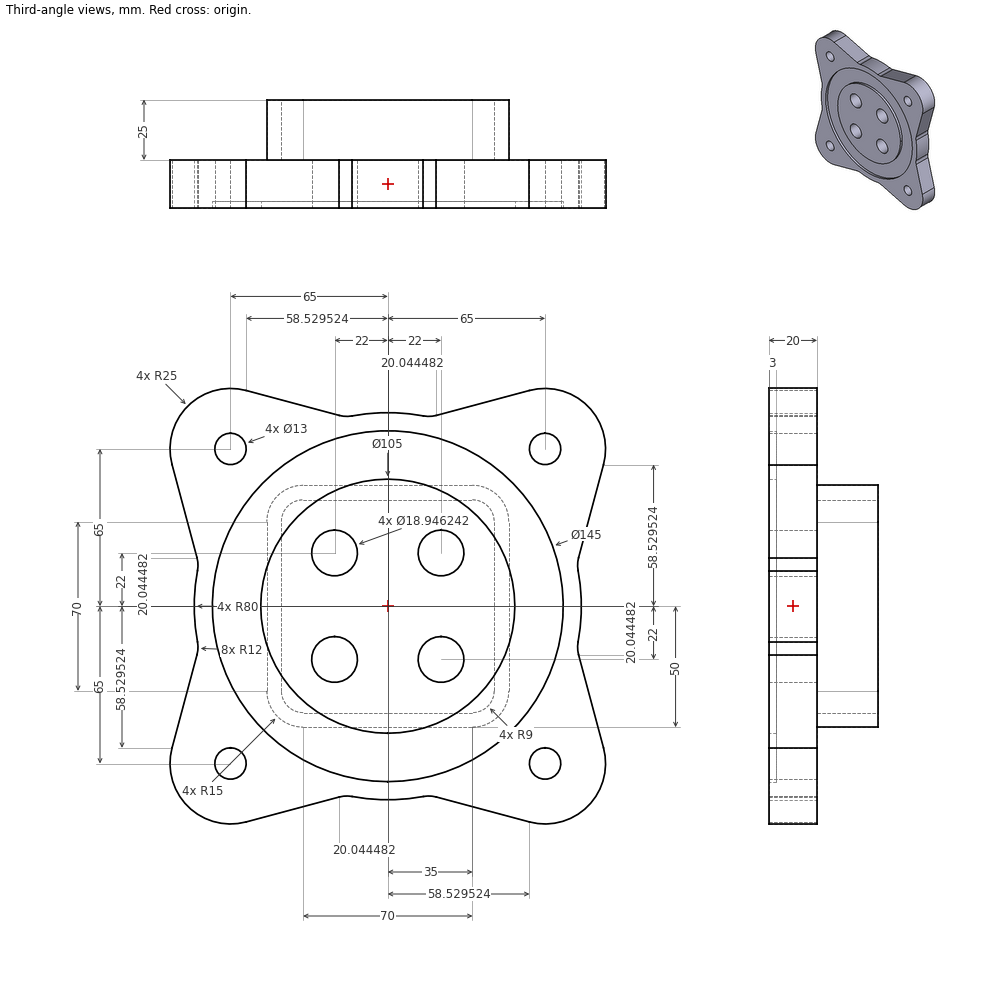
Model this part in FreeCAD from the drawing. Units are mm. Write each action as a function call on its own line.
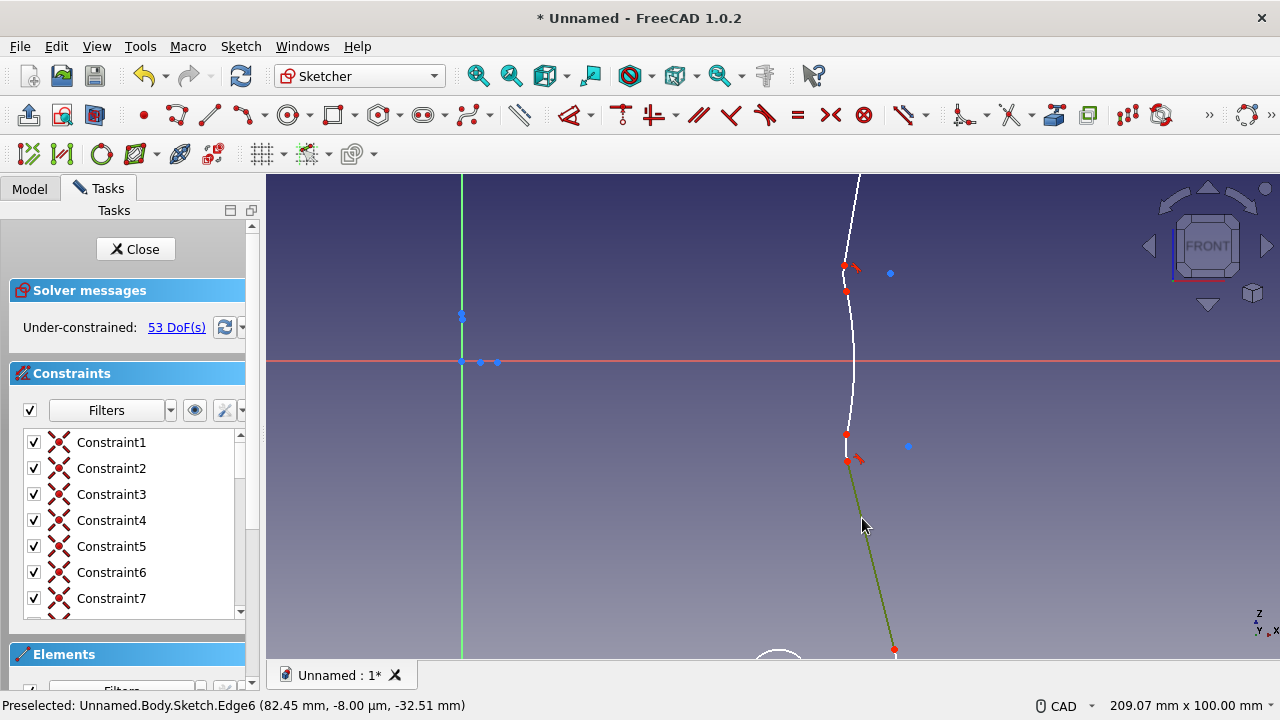
scroll(846, 449, down, 5)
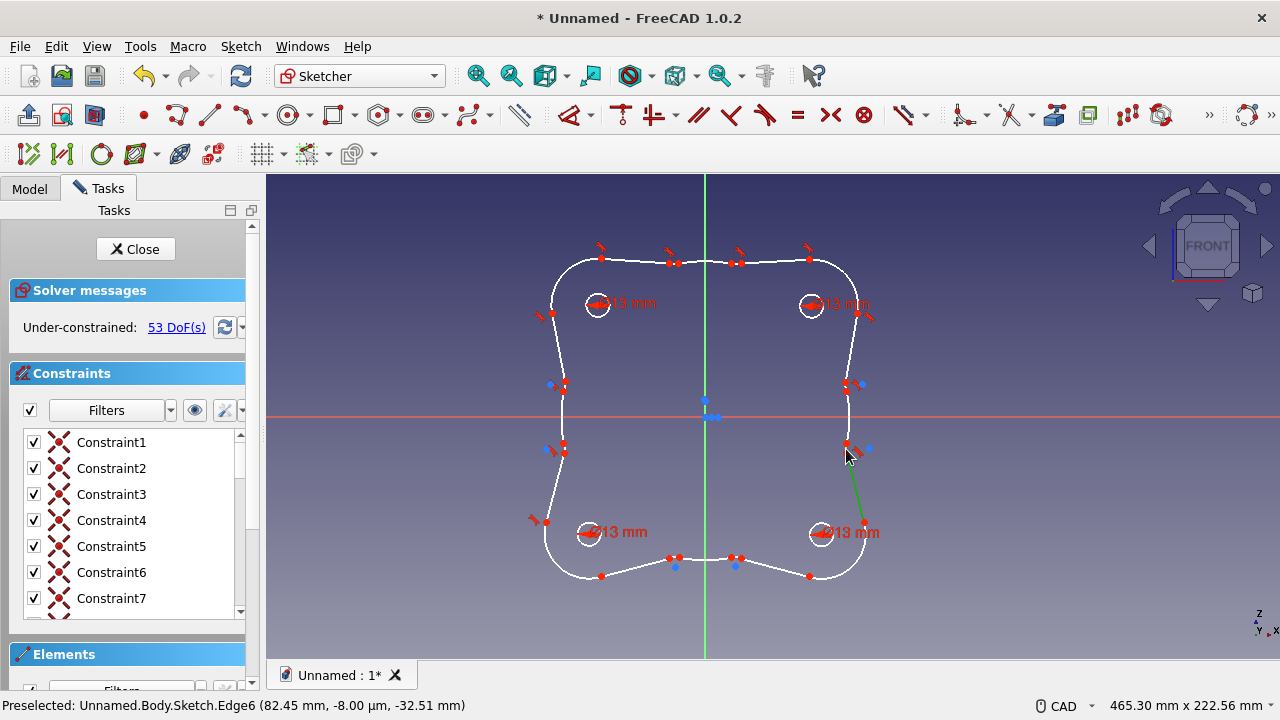
click(837, 576)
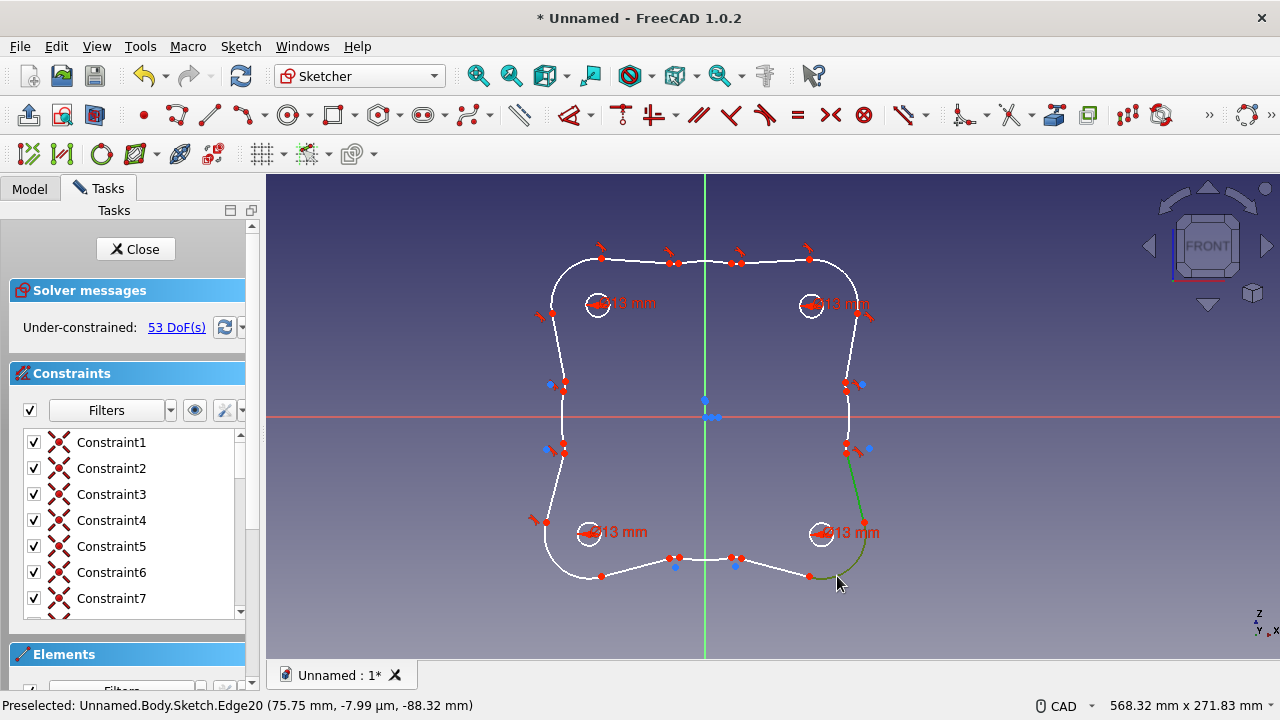
click(765, 116)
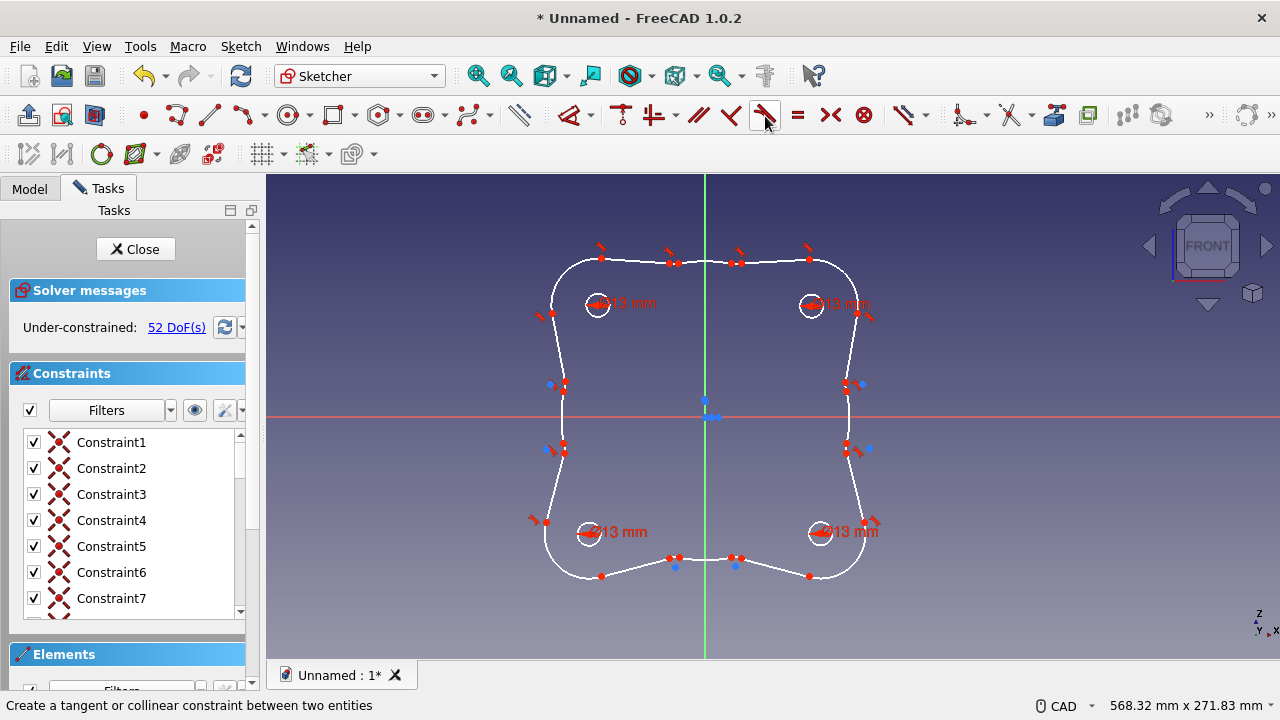
click(789, 572)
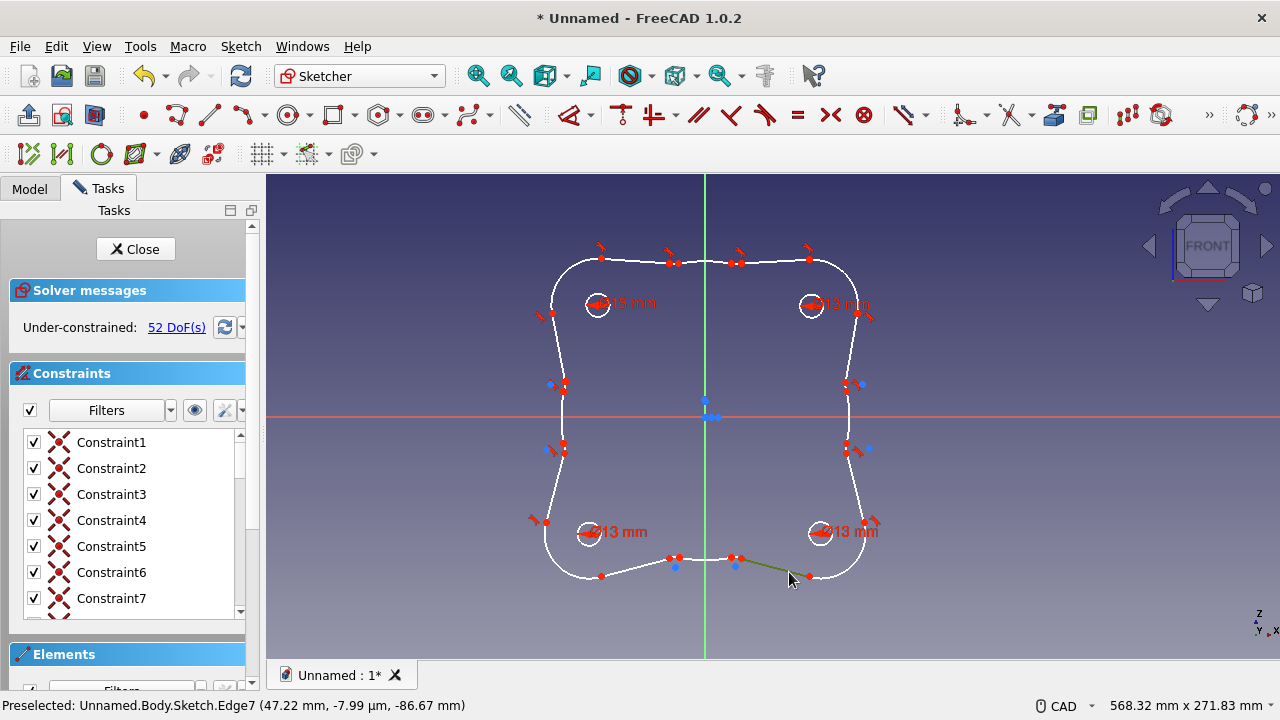
click(836, 576)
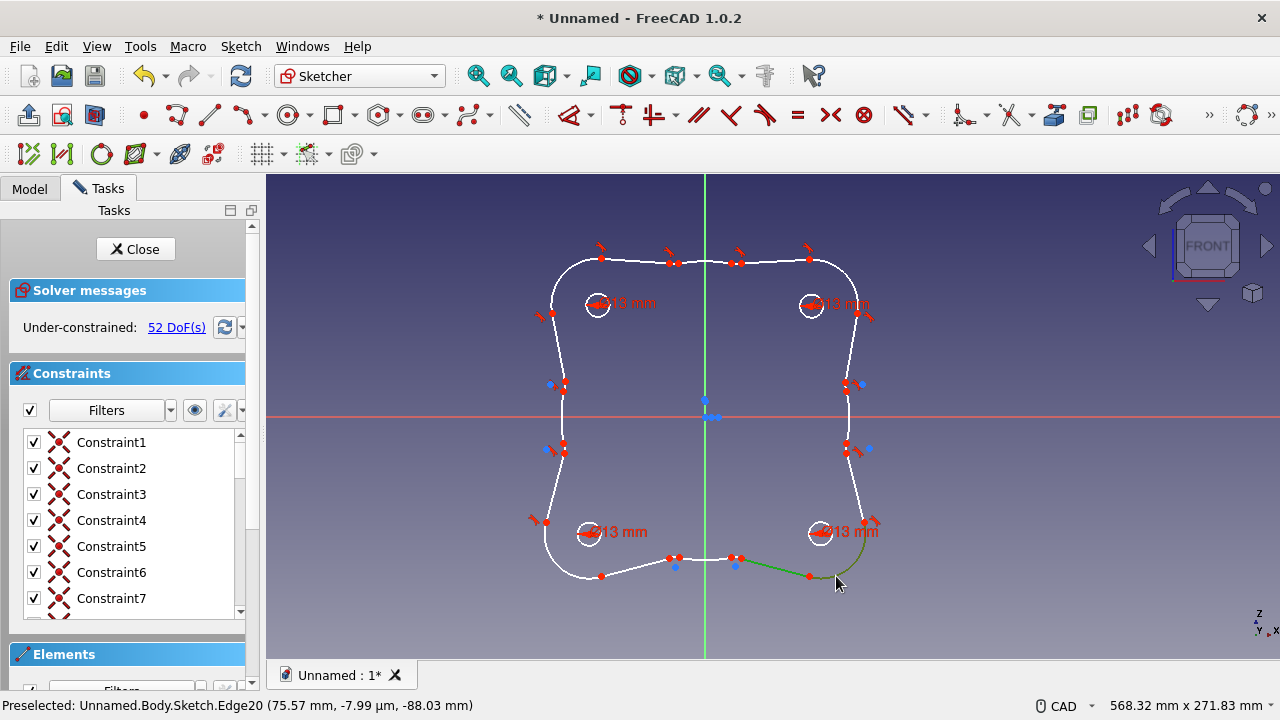
click(765, 116)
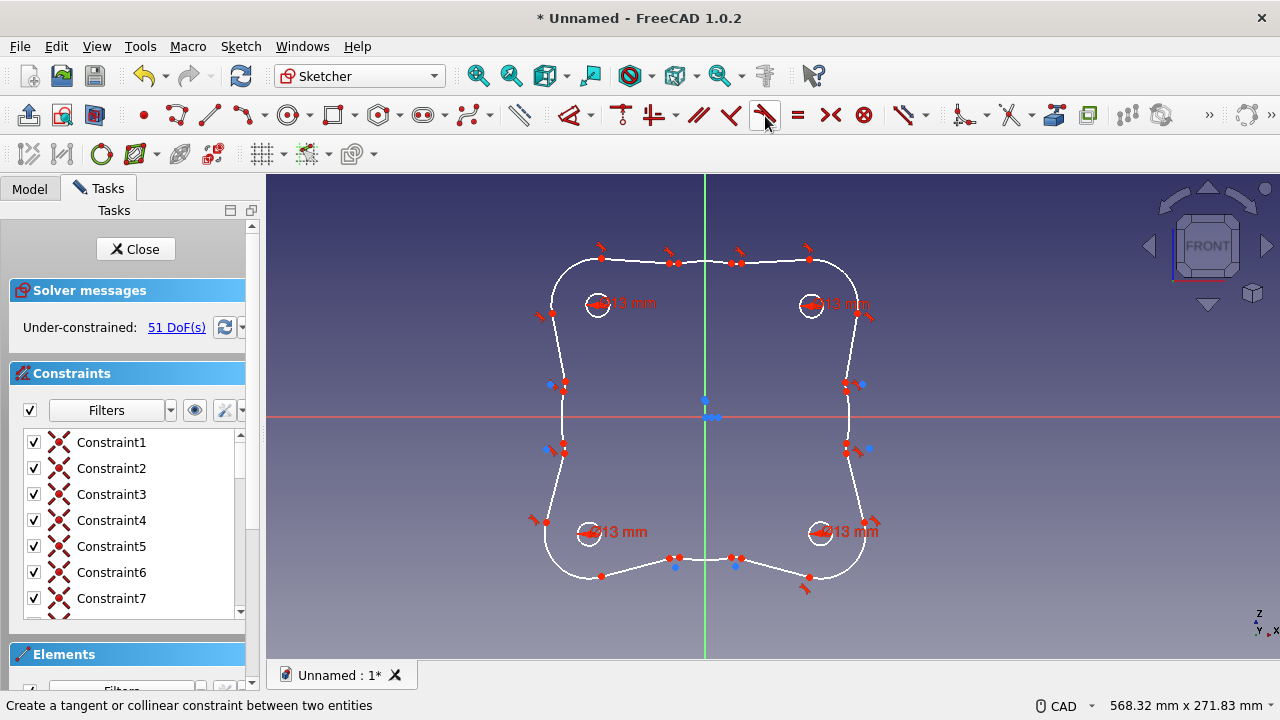
click(789, 572)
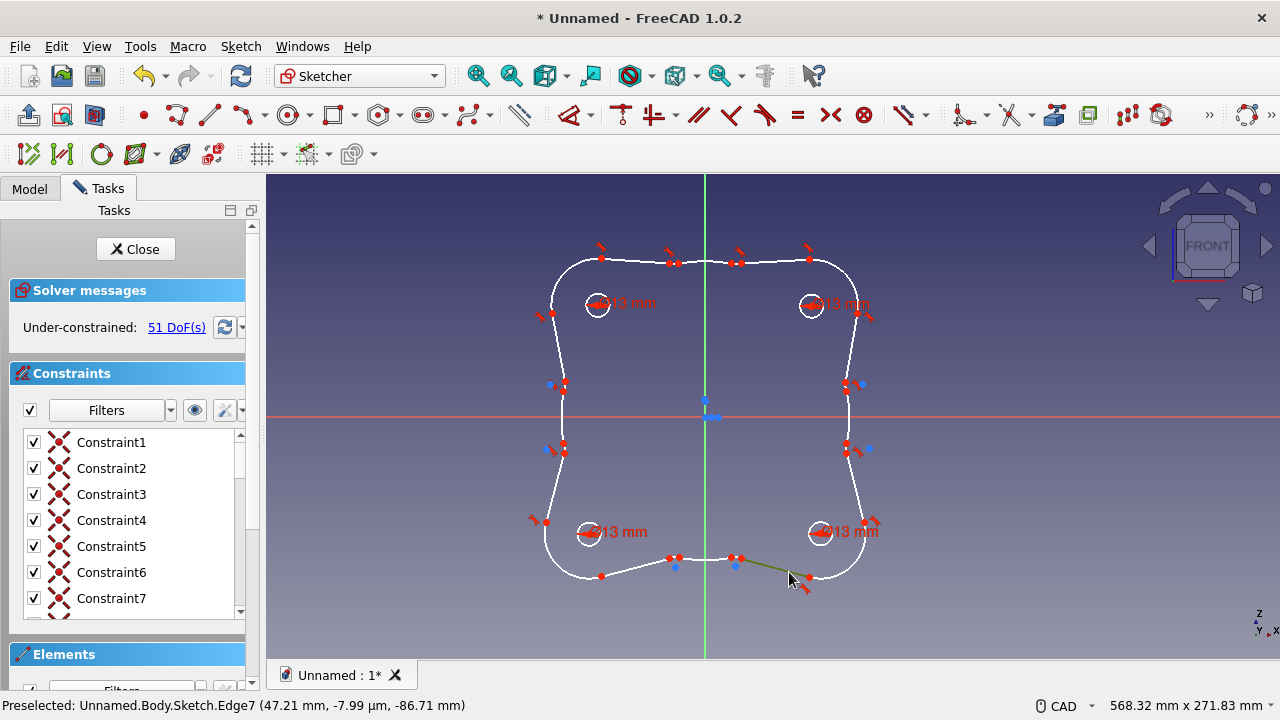
scroll(736, 557, up, 6)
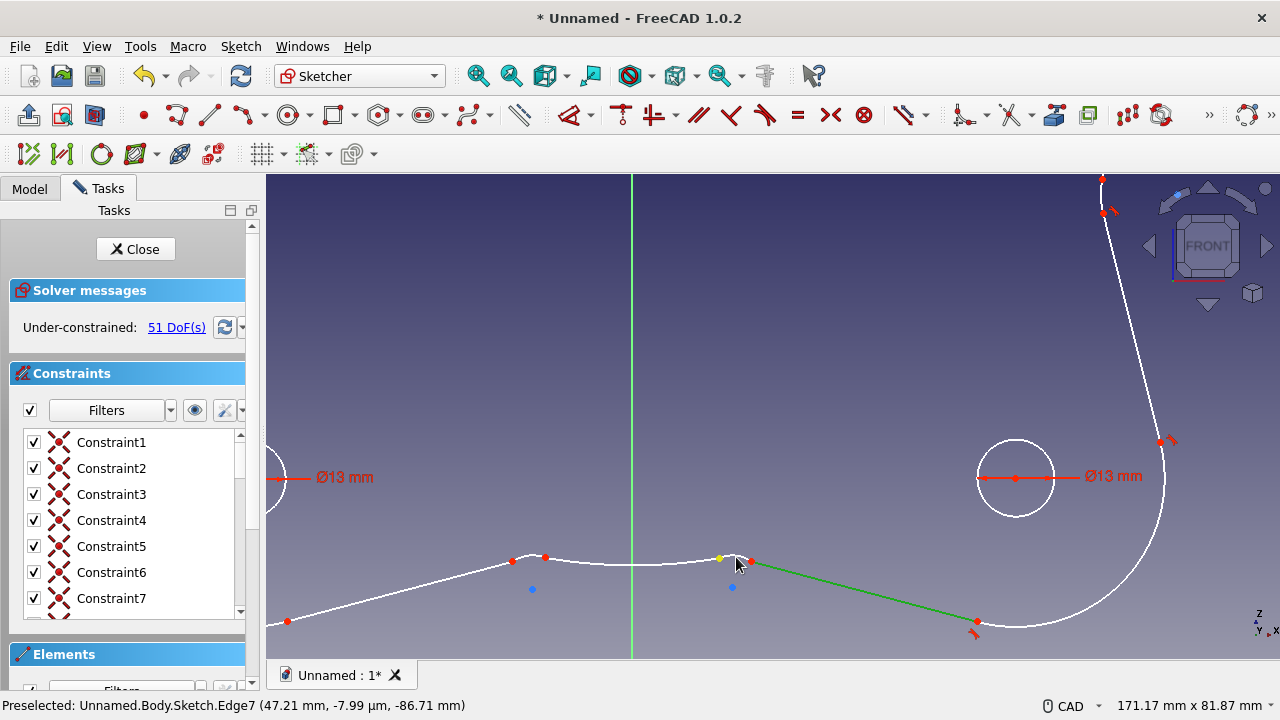
click(736, 556)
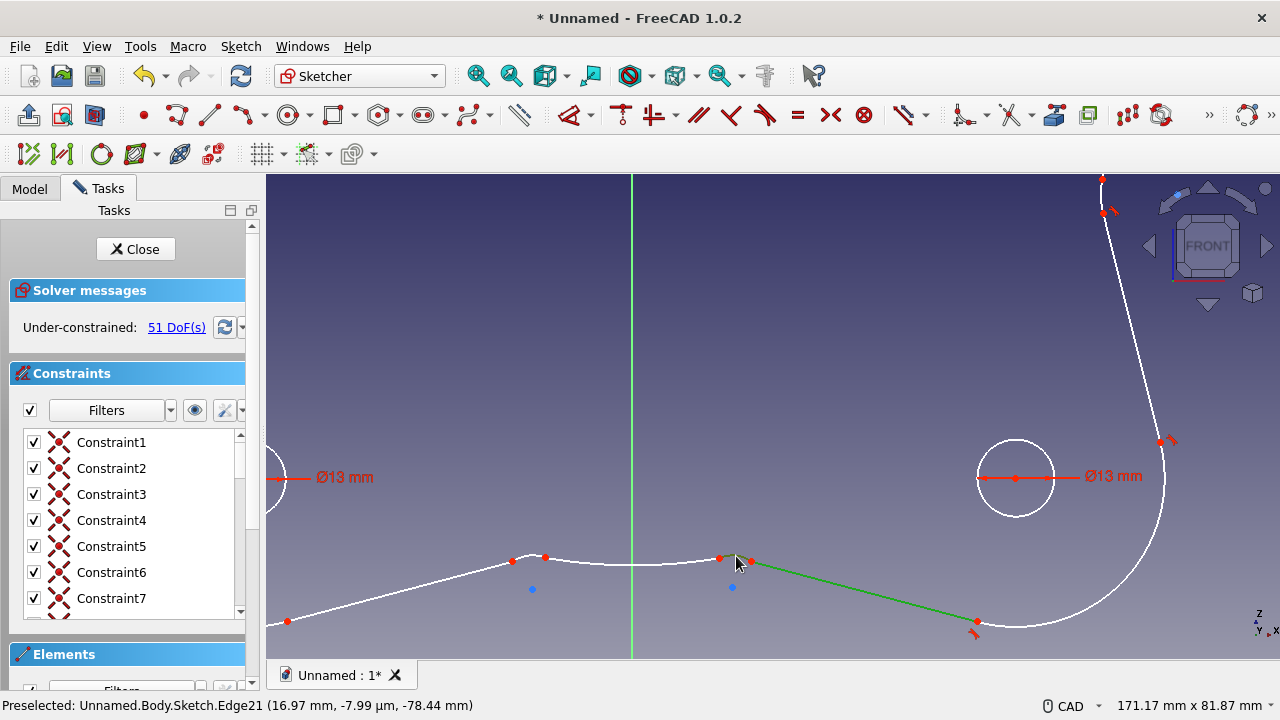
click(765, 116)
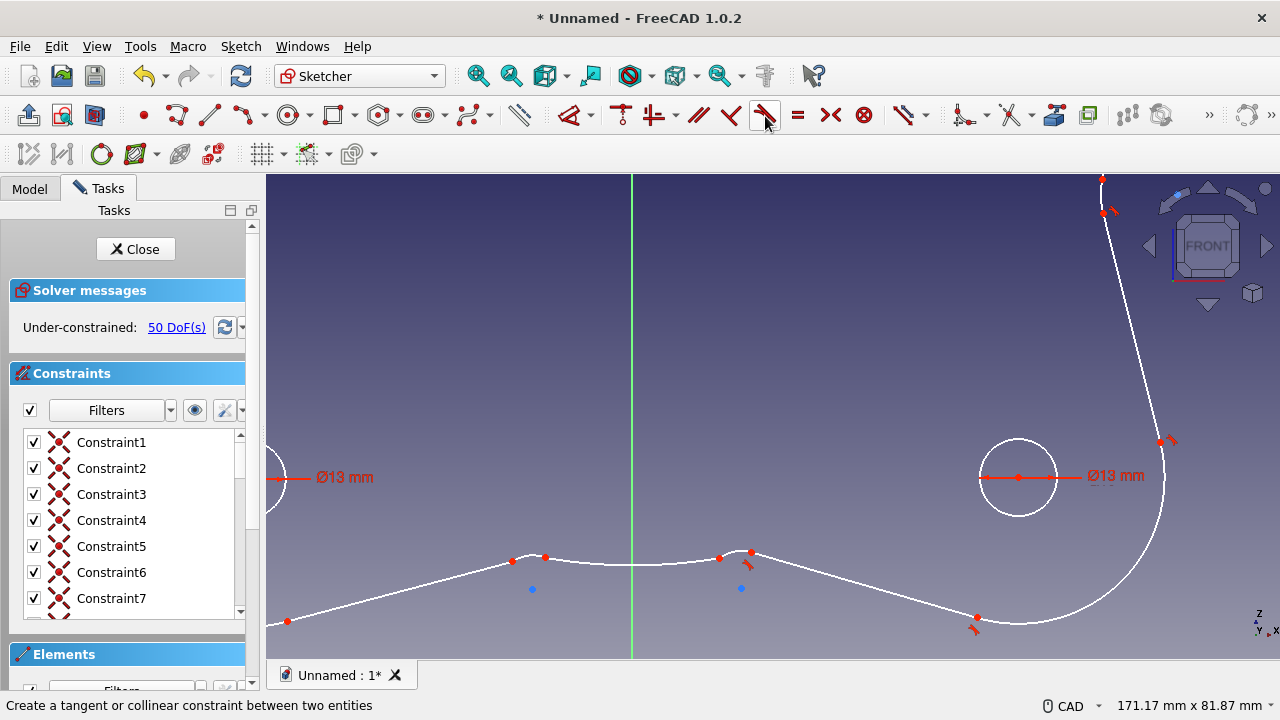
click(445, 580)